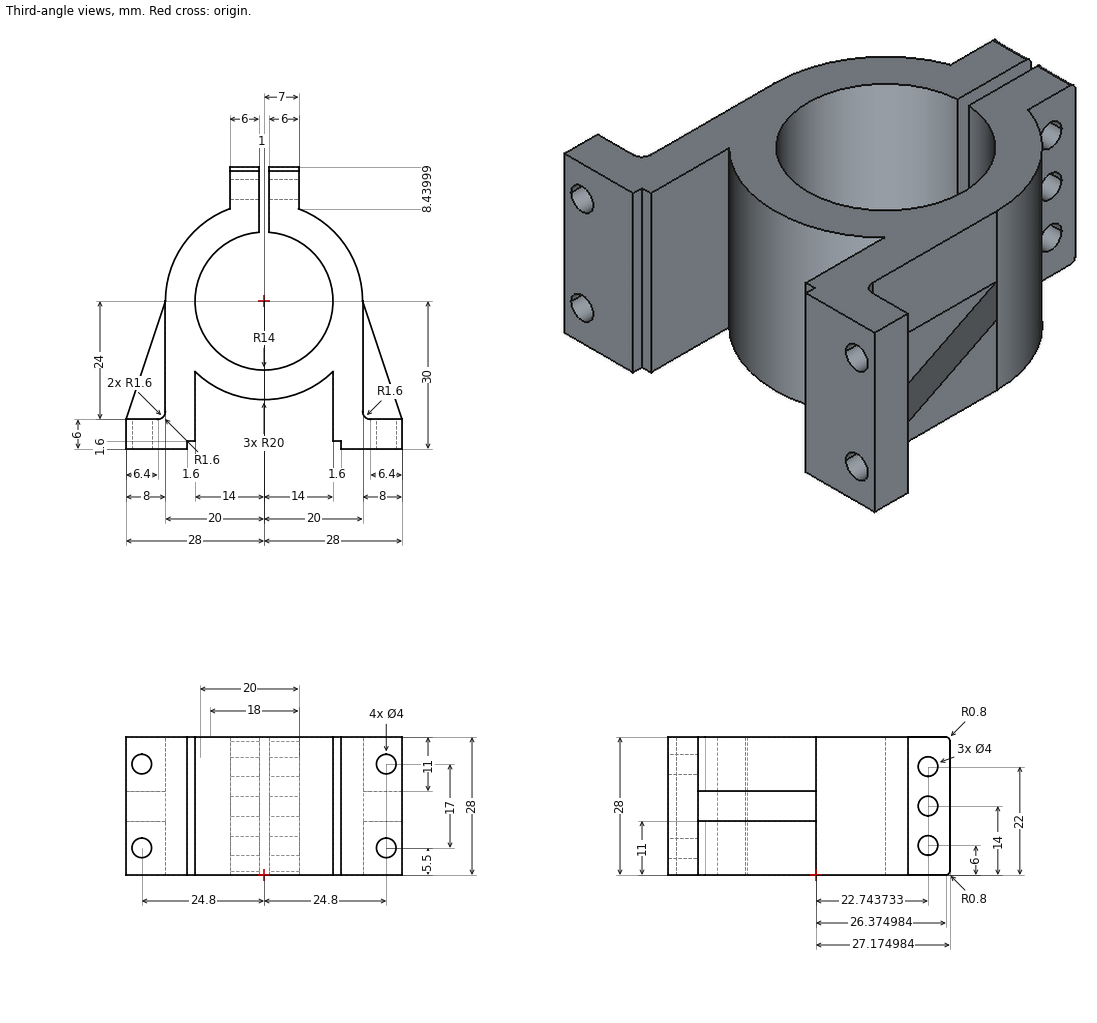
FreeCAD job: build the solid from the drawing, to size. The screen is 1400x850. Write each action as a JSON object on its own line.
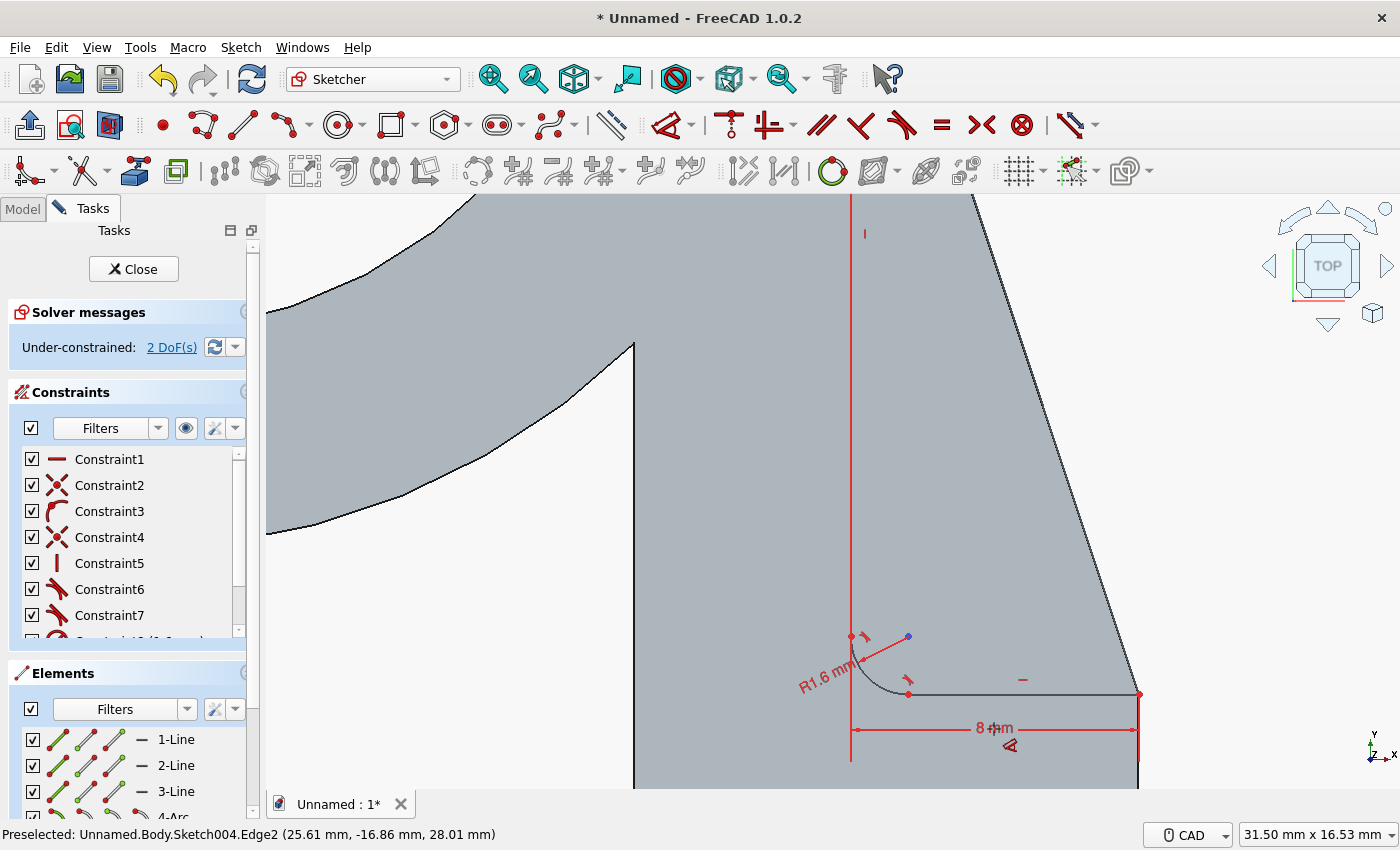
{"action": "left_click", "coordinate": [909, 695]}
{"action": "left_click", "coordinate": [943, 458]}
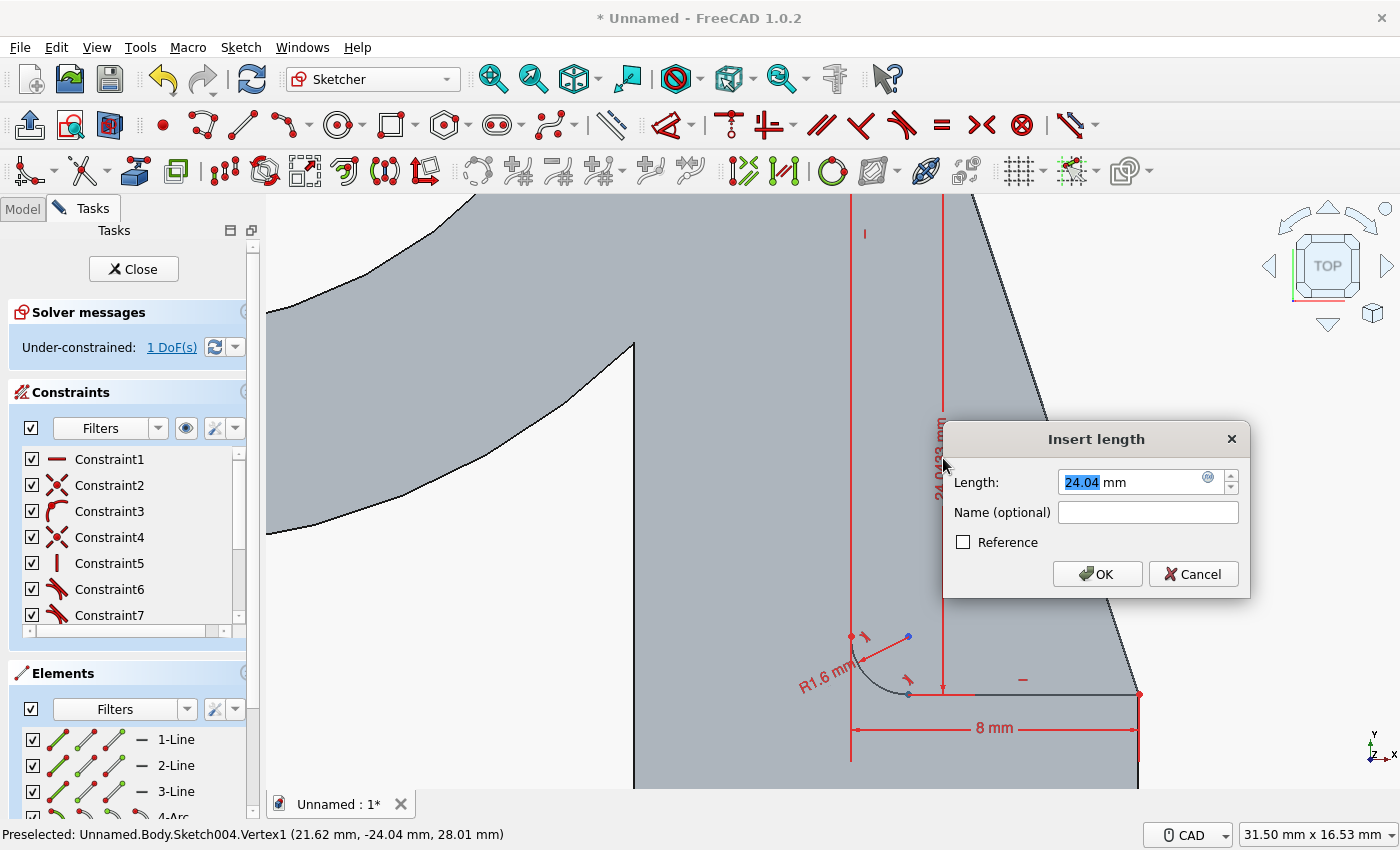
{"action": "type", "text": "24"}
{"action": "key", "text": "Return"}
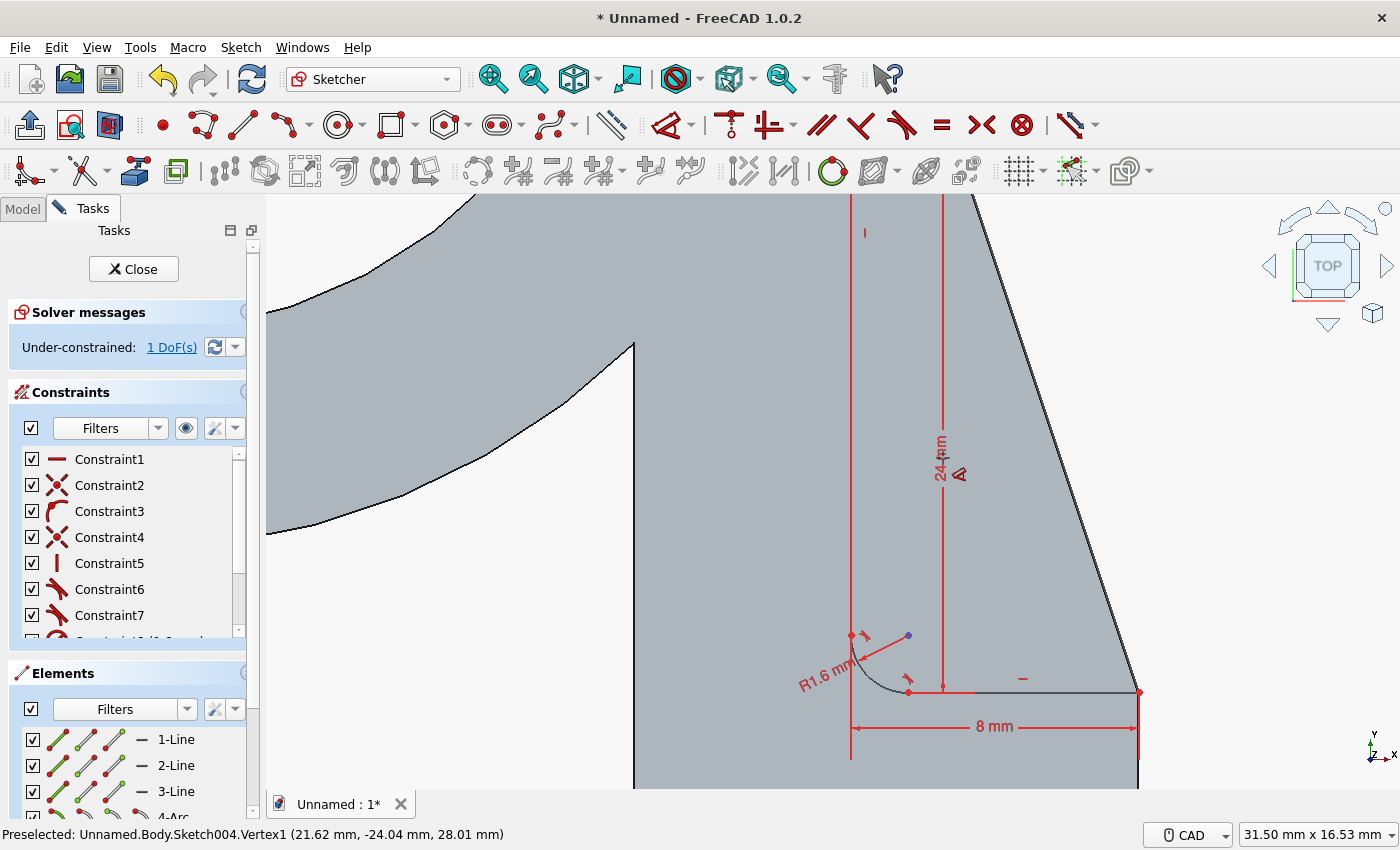
{"action": "left_click", "coordinate": [1139, 693]}
{"action": "left_click", "coordinate": [717, 727]}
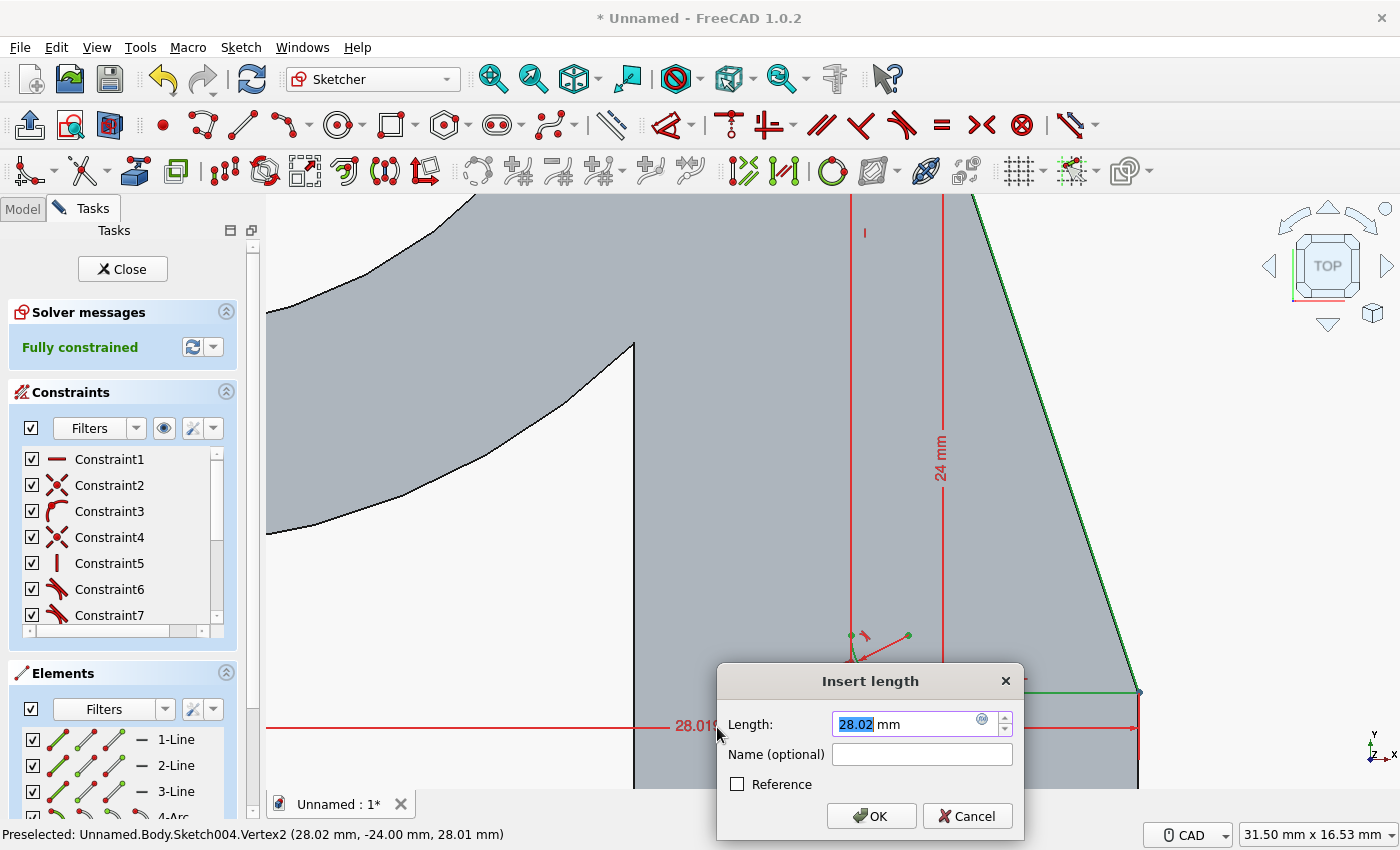
{"action": "type", "text": "28"}
{"action": "key", "text": "Return"}
{"action": "key", "text": "Escape"}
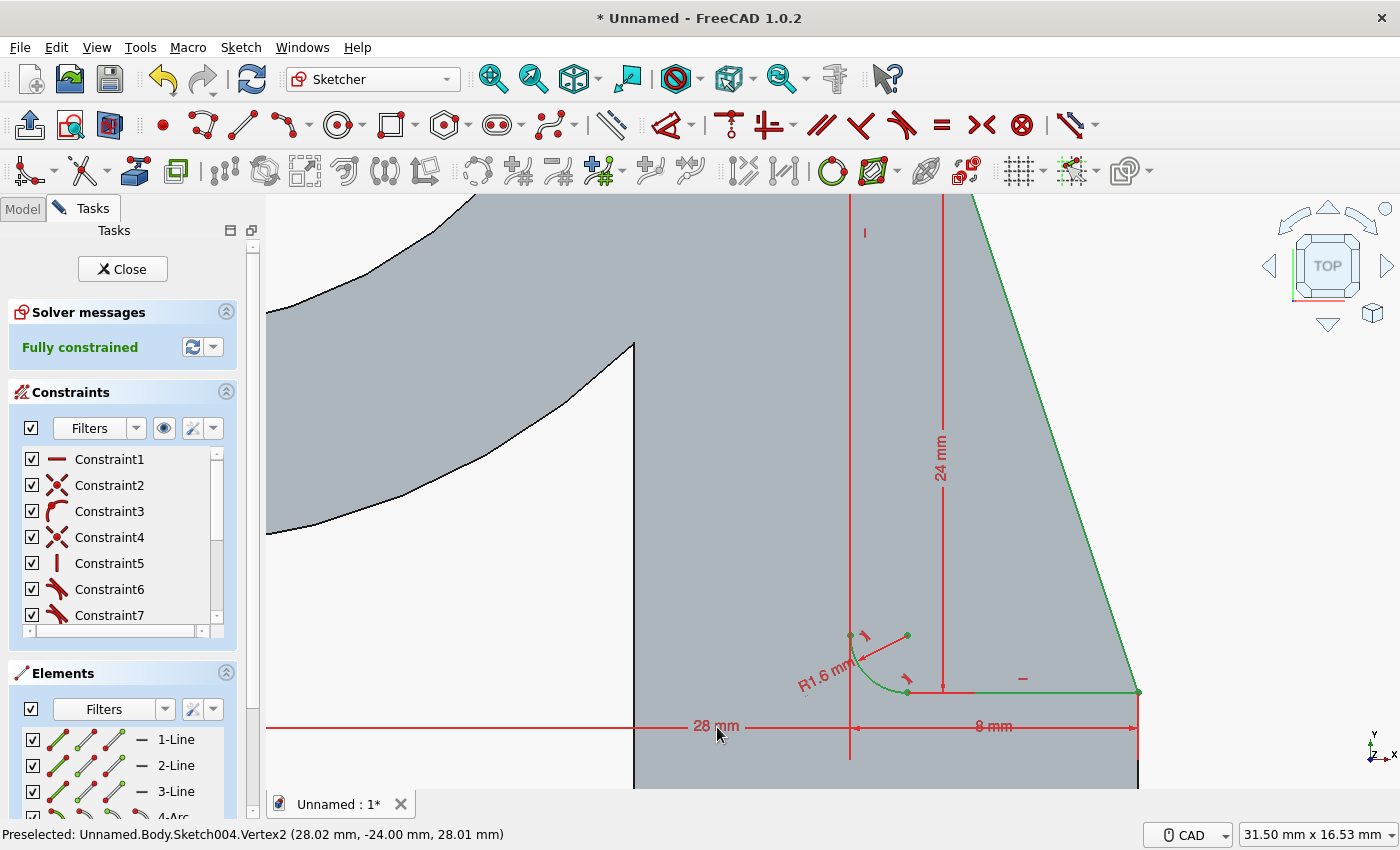
{"action": "left_click", "coordinate": [123, 269]}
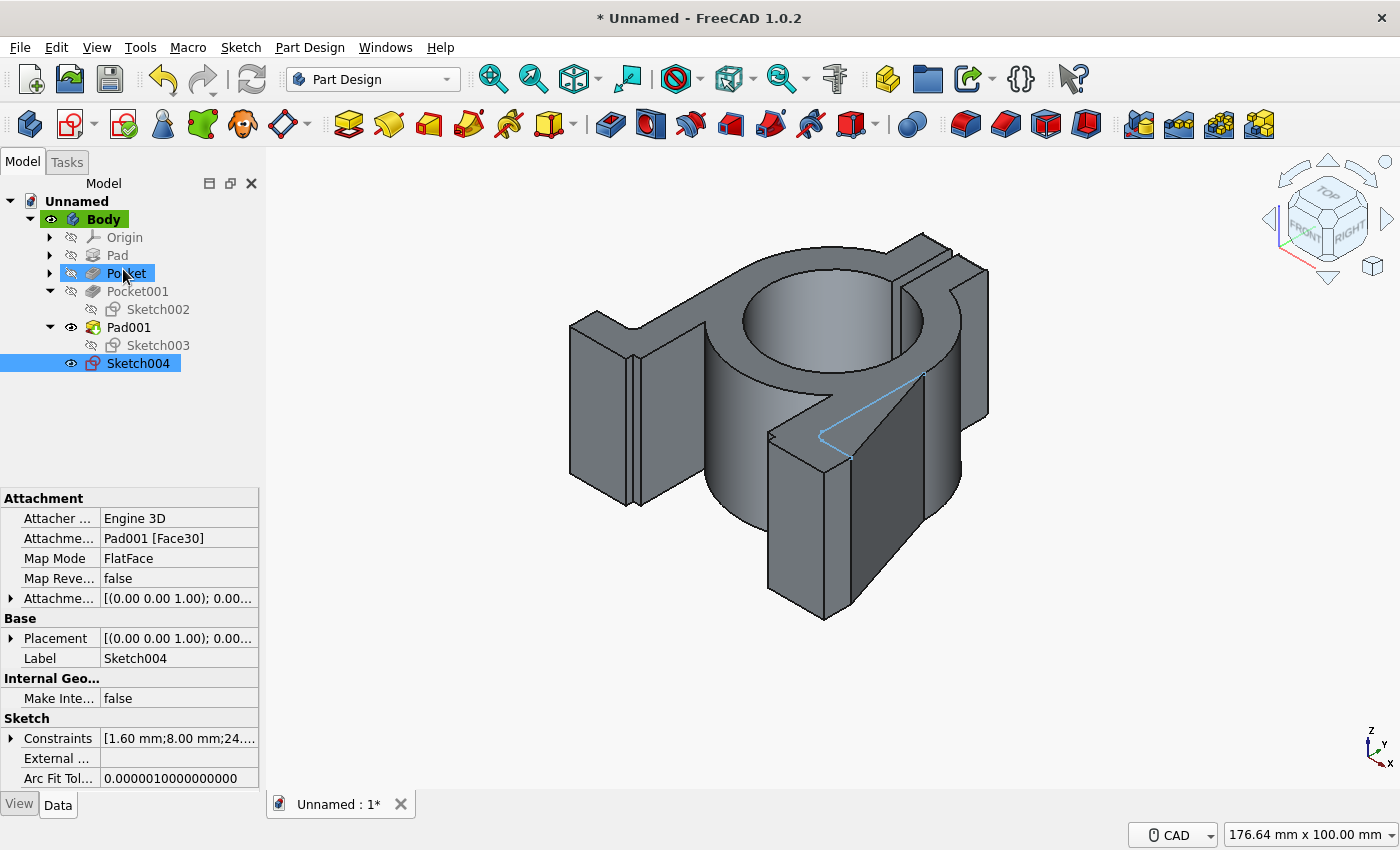
{"action": "left_click", "coordinate": [612, 124]}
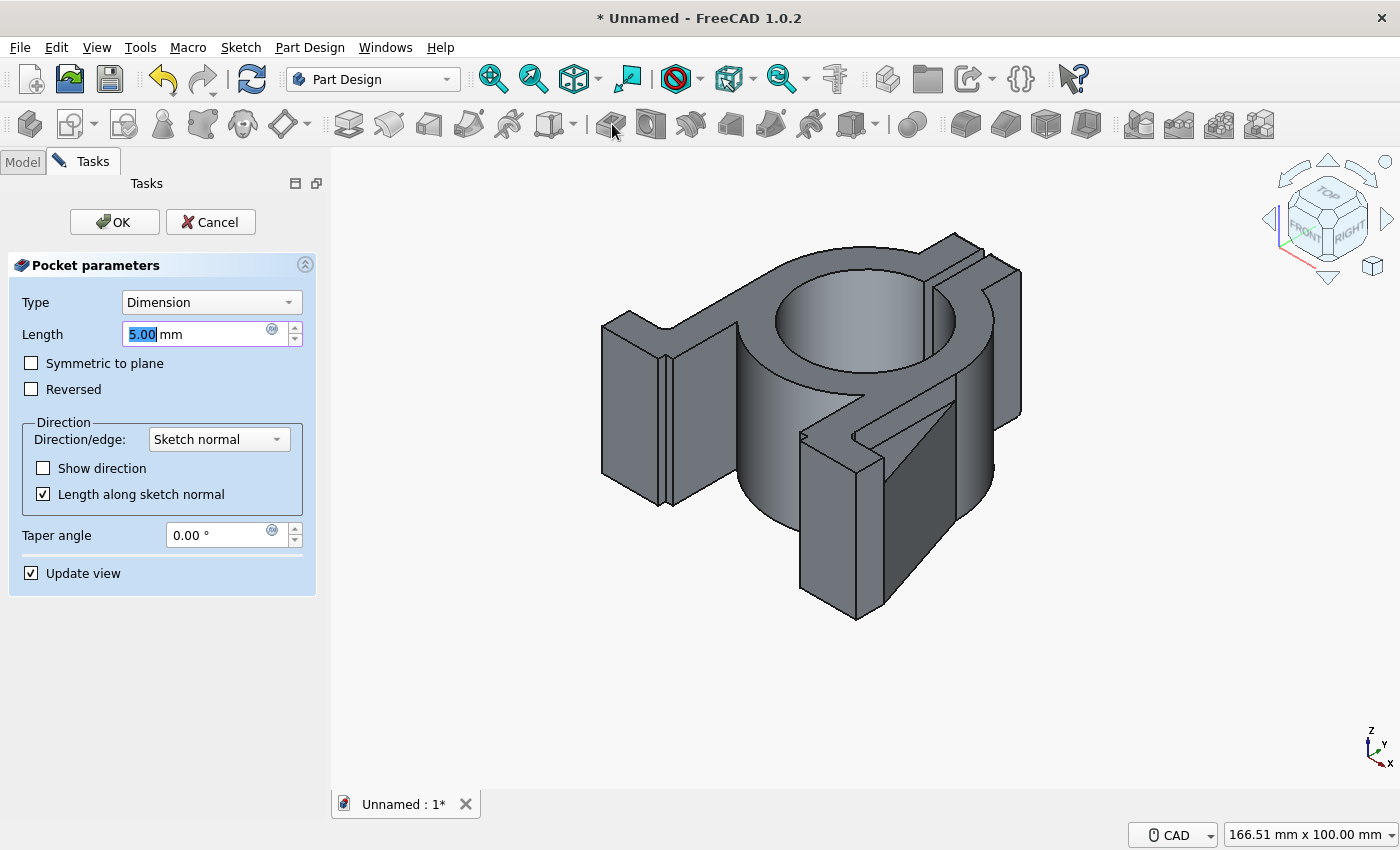
{"action": "type", "text": "11"}
{"action": "key", "text": "Tab"}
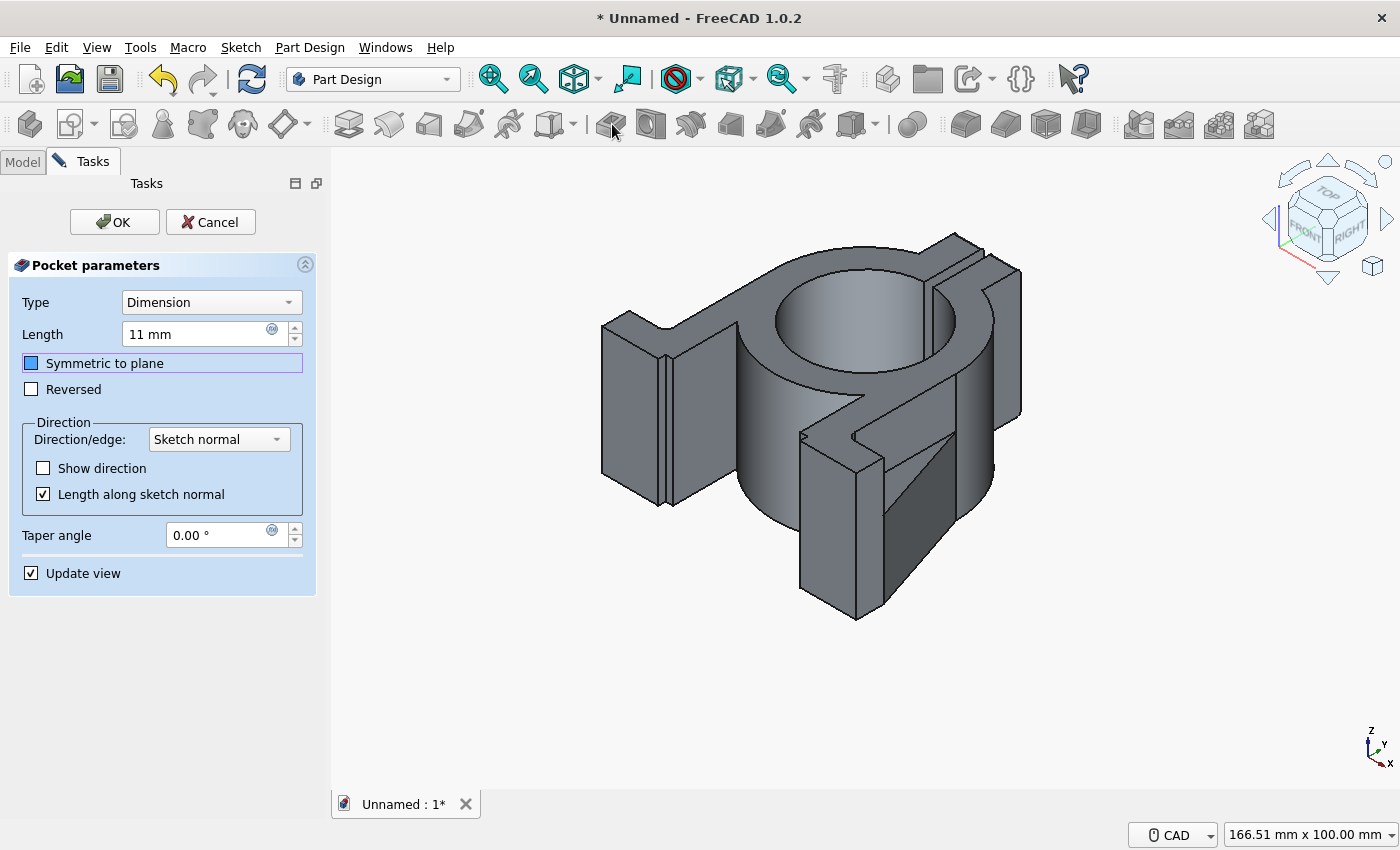
{"action": "left_click", "coordinate": [115, 222]}